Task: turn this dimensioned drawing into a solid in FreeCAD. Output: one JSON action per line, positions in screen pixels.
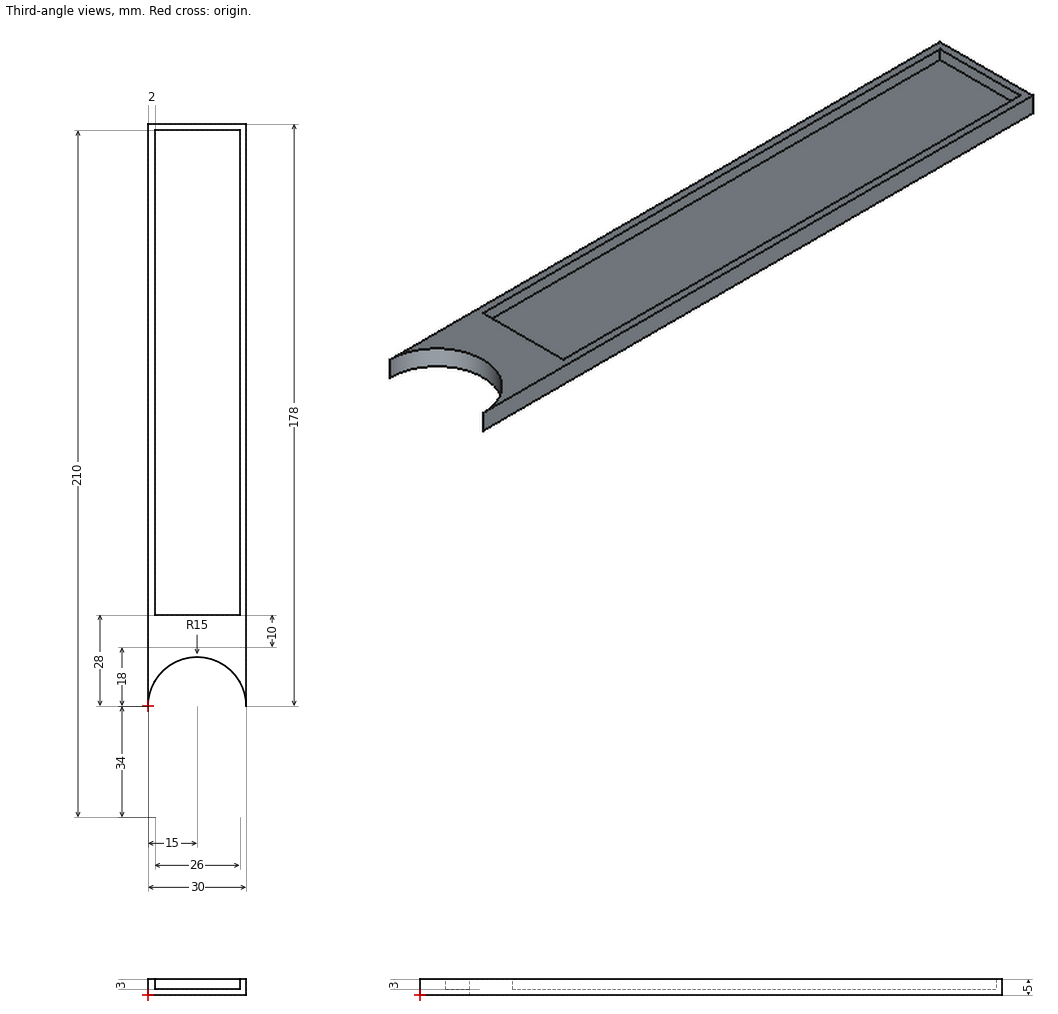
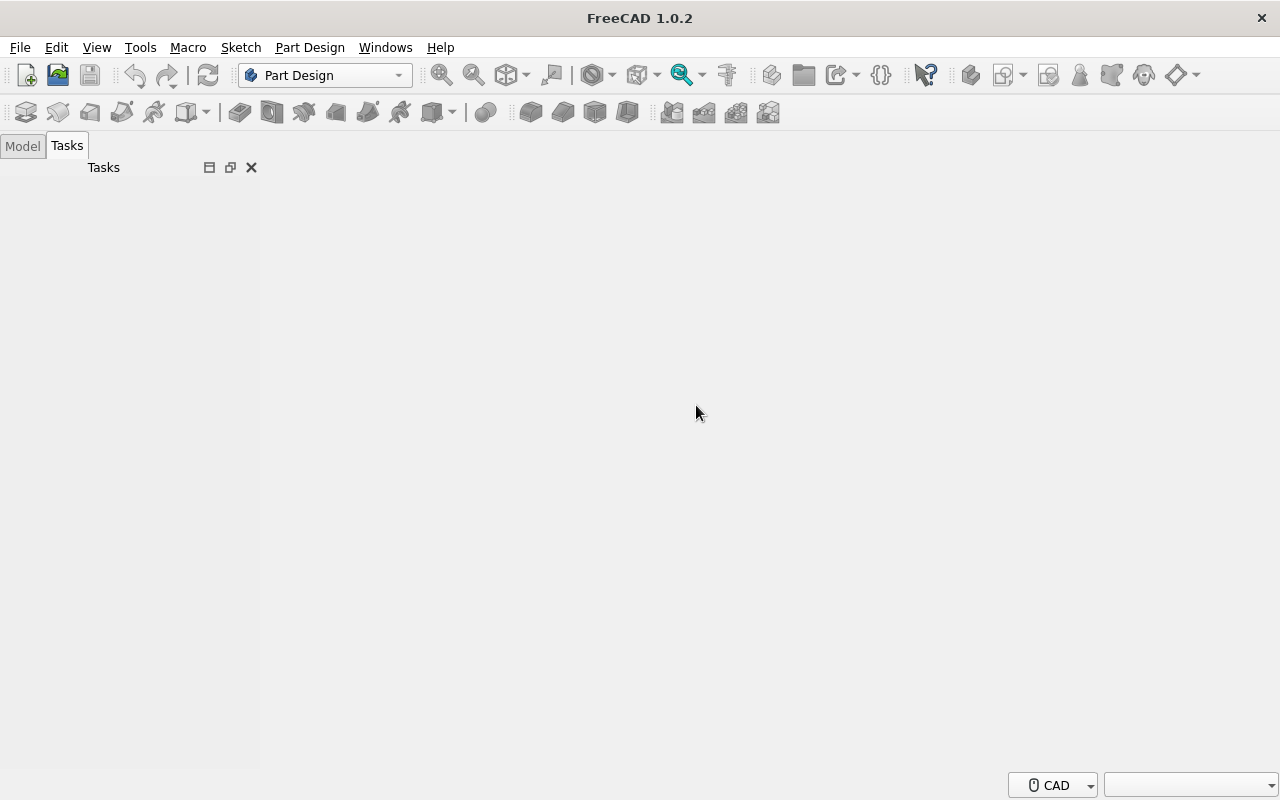
{"action": "key", "text": "ctrl+n"}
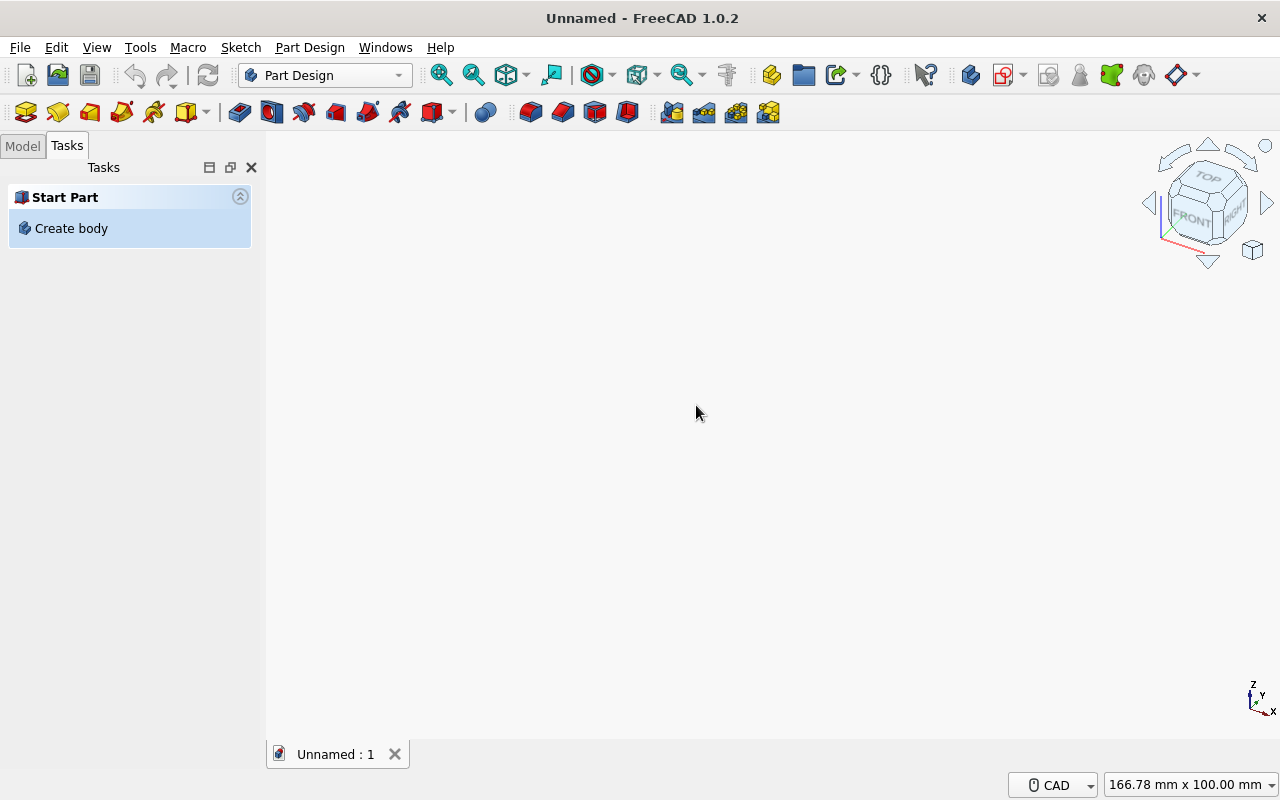
{"action": "left_click", "coordinate": [1004, 76]}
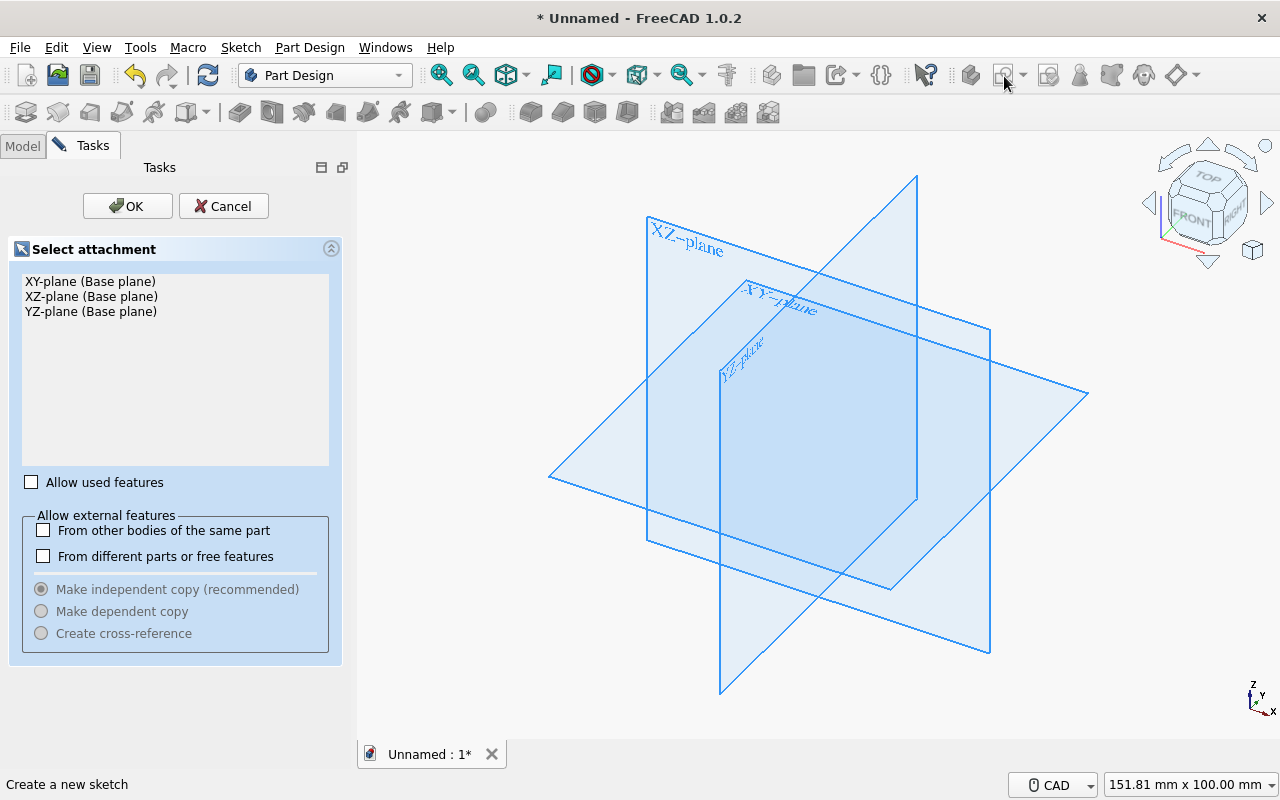
{"action": "left_click", "coordinate": [82, 282]}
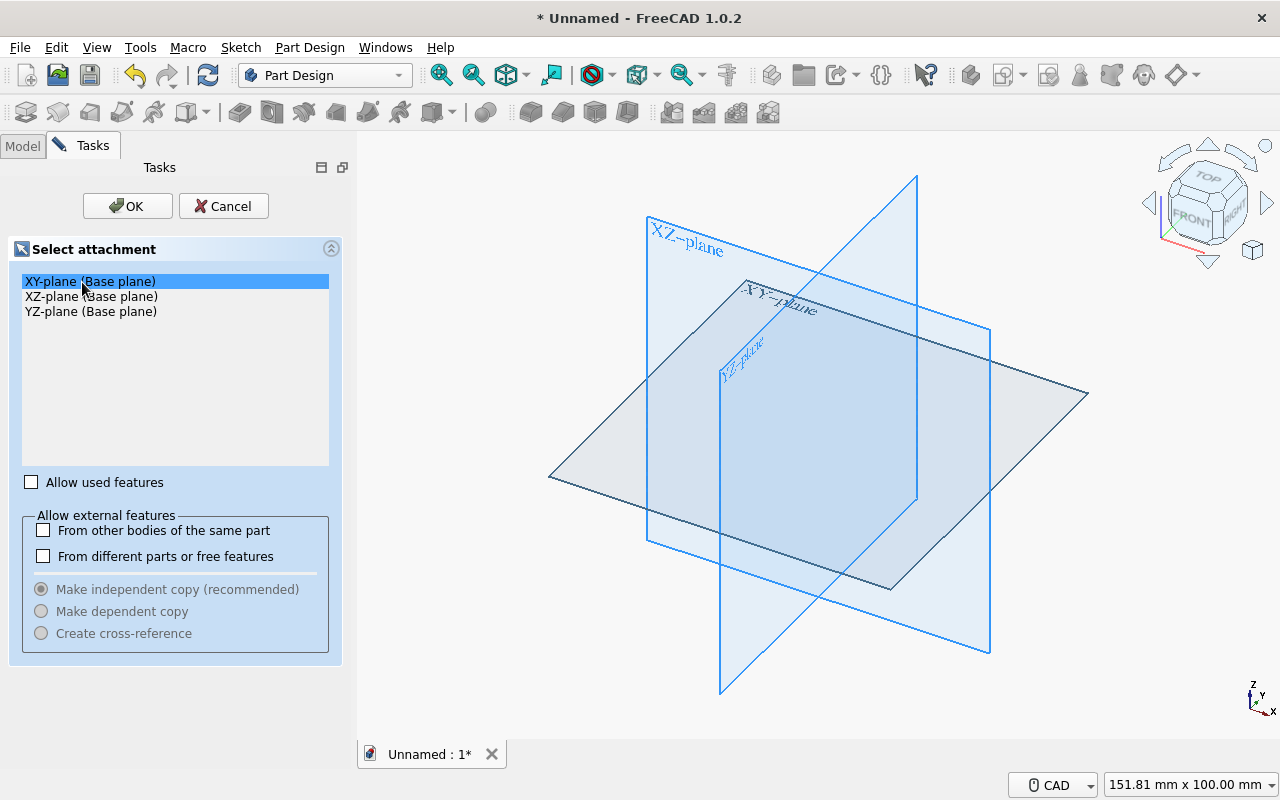
{"action": "left_click", "coordinate": [128, 206]}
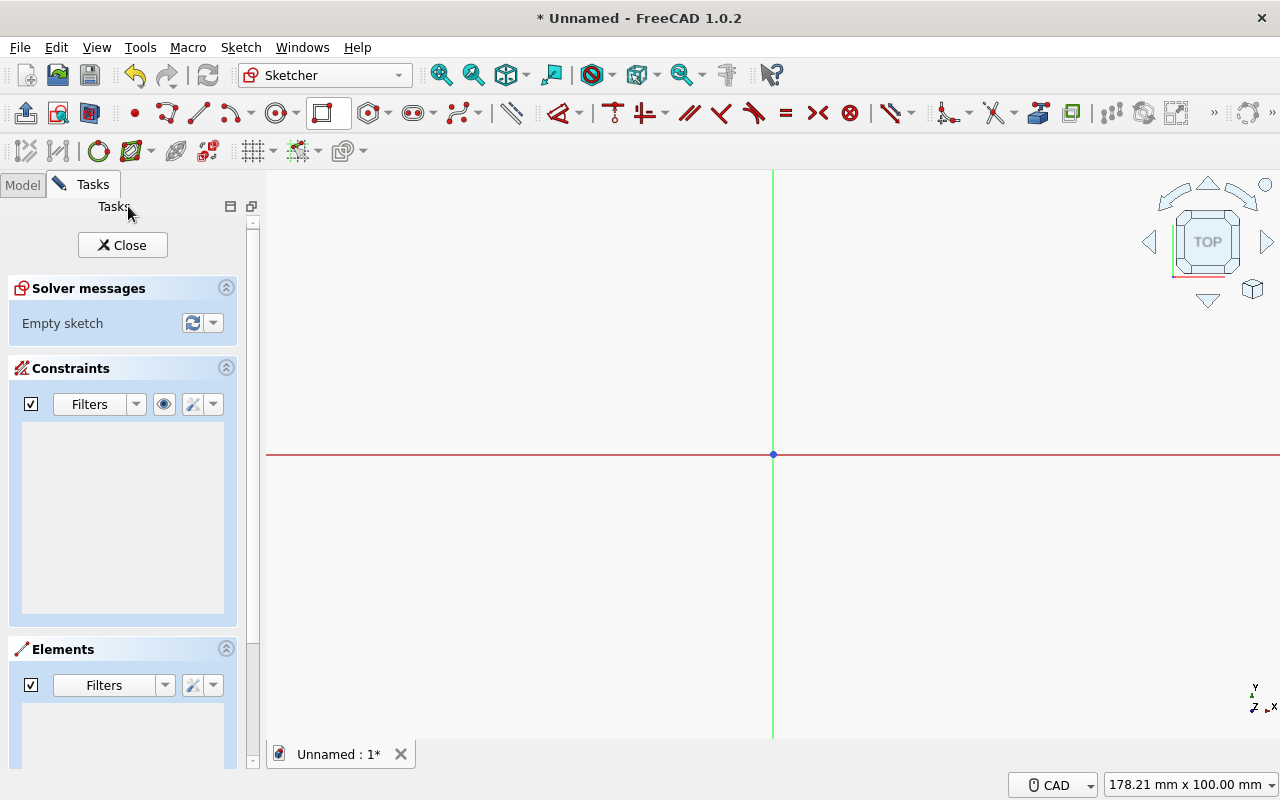
{"action": "scroll", "coordinate": [615, 711], "scroll_direction": "down", "scroll_amount": 5}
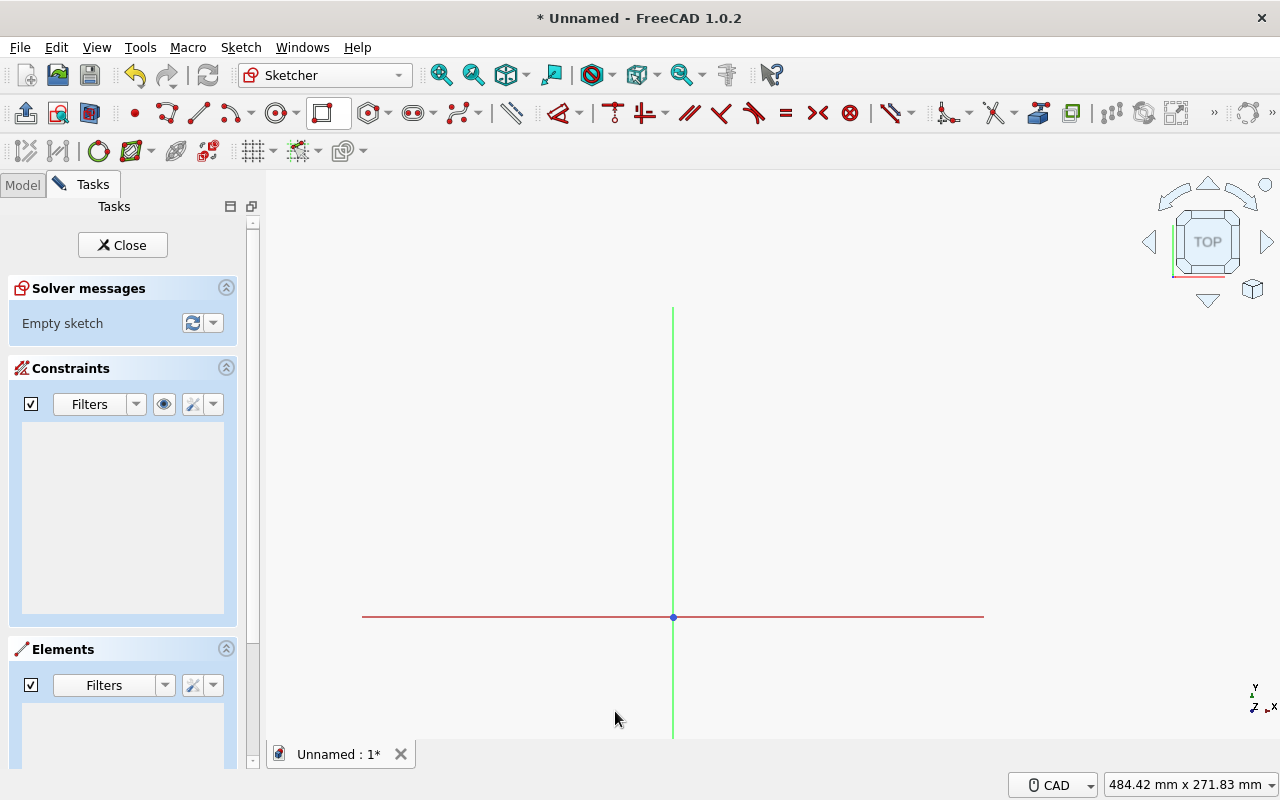
{"action": "key", "text": "g r"}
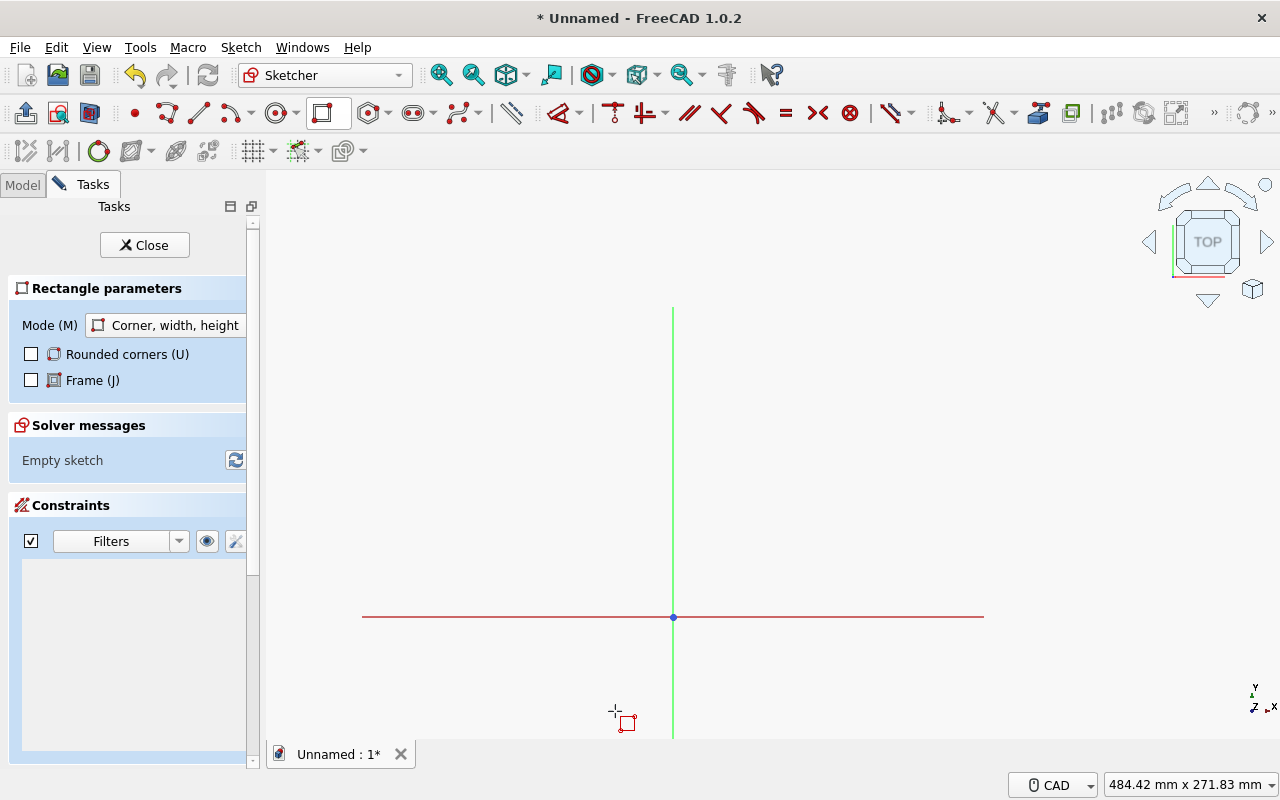
{"action": "left_click", "coordinate": [673, 617]}
{"action": "mouse_move", "coordinate": [736, 245]}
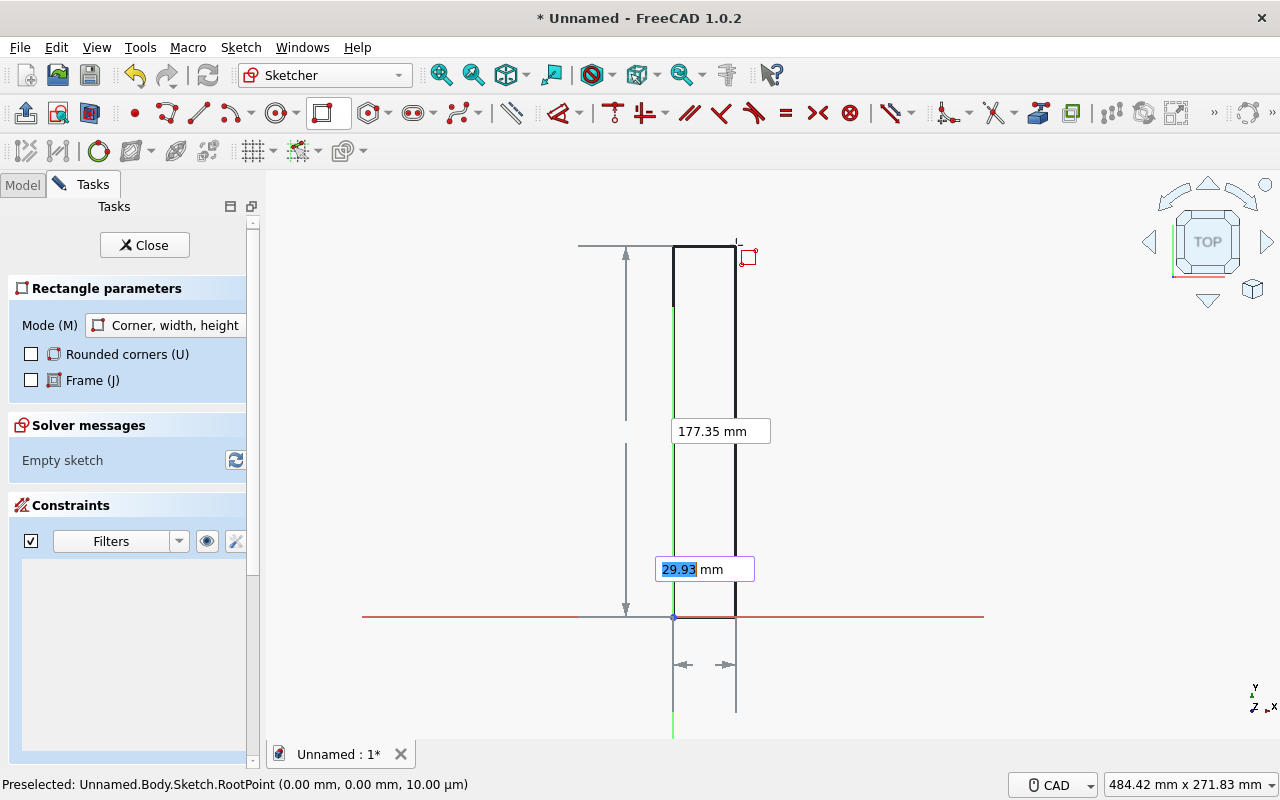
{"action": "type", "text": "30"}
{"action": "key", "text": "Tab"}
{"action": "type", "text": "178"}
{"action": "key", "text": "Return"}
{"action": "key", "text": "Escape"}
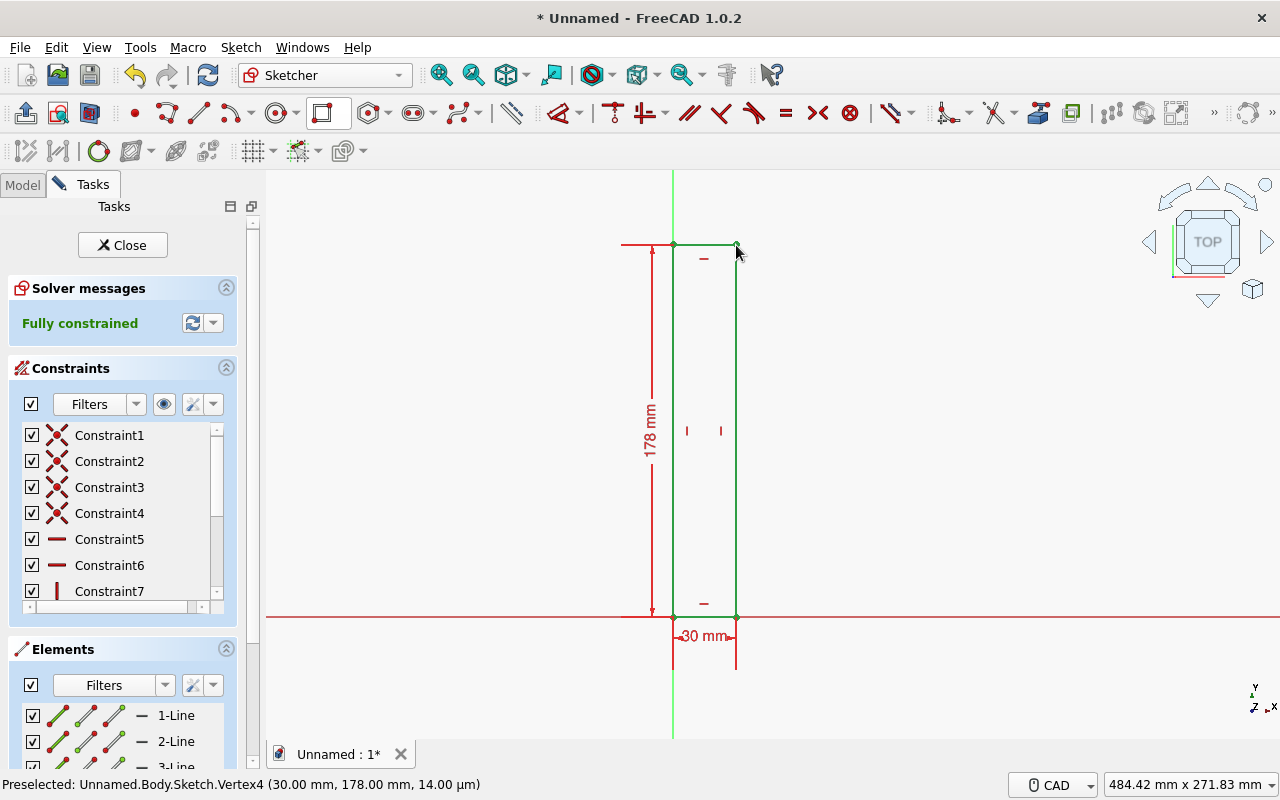
{"action": "left_click", "coordinate": [123, 245]}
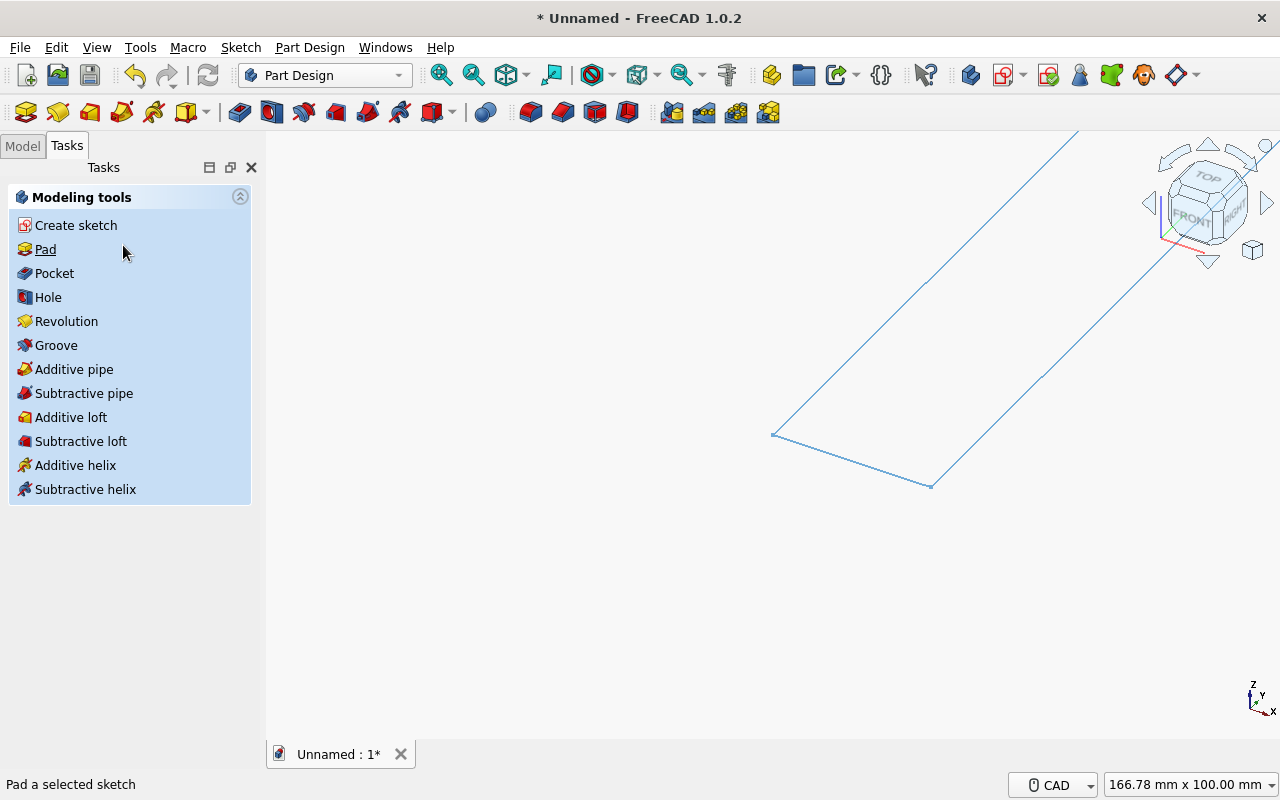
{"action": "left_click", "coordinate": [26, 112]}